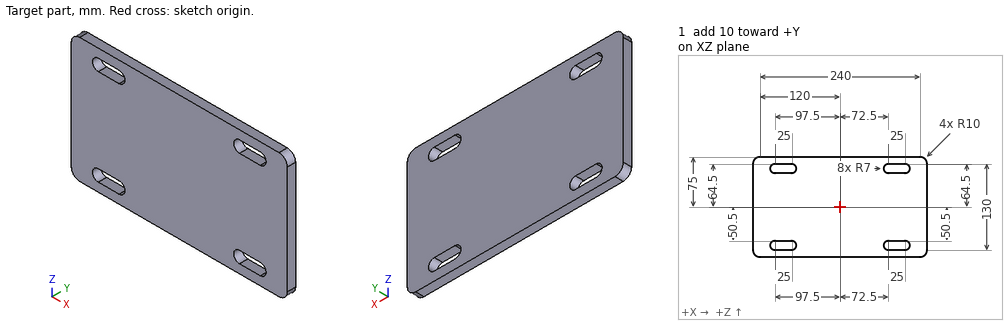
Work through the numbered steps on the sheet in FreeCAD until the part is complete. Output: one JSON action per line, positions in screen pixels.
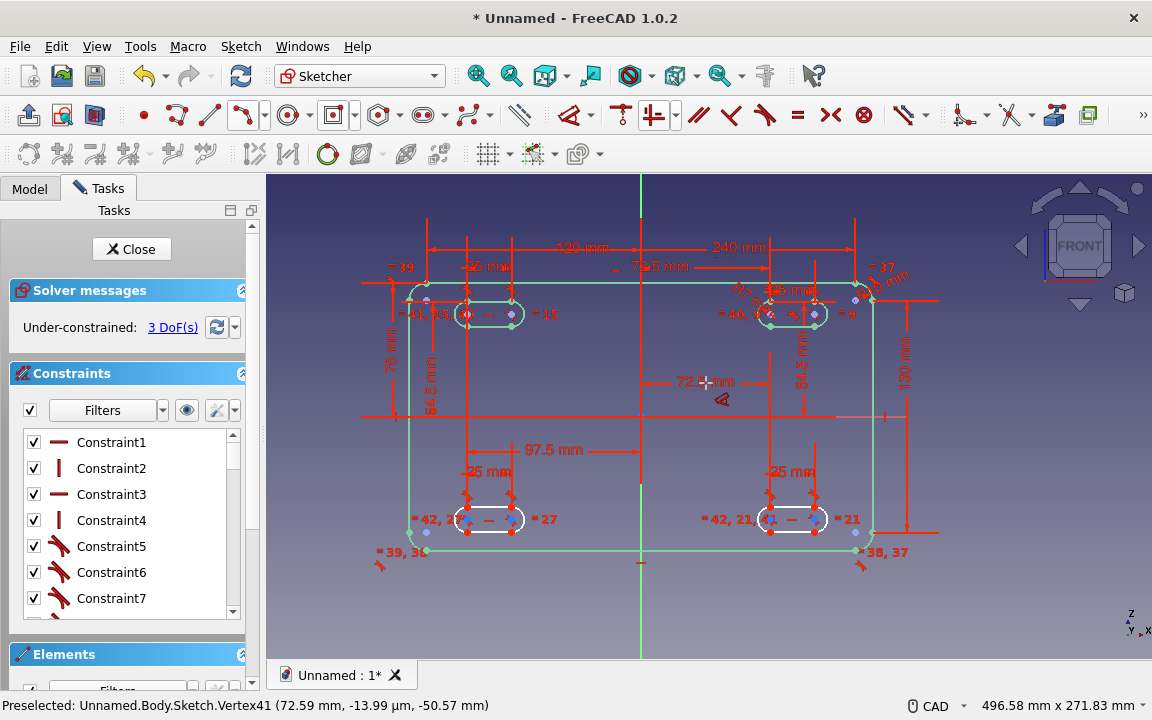
{"action": "left_click", "coordinate": [770, 507]}
{"action": "left_click", "coordinate": [804, 441]}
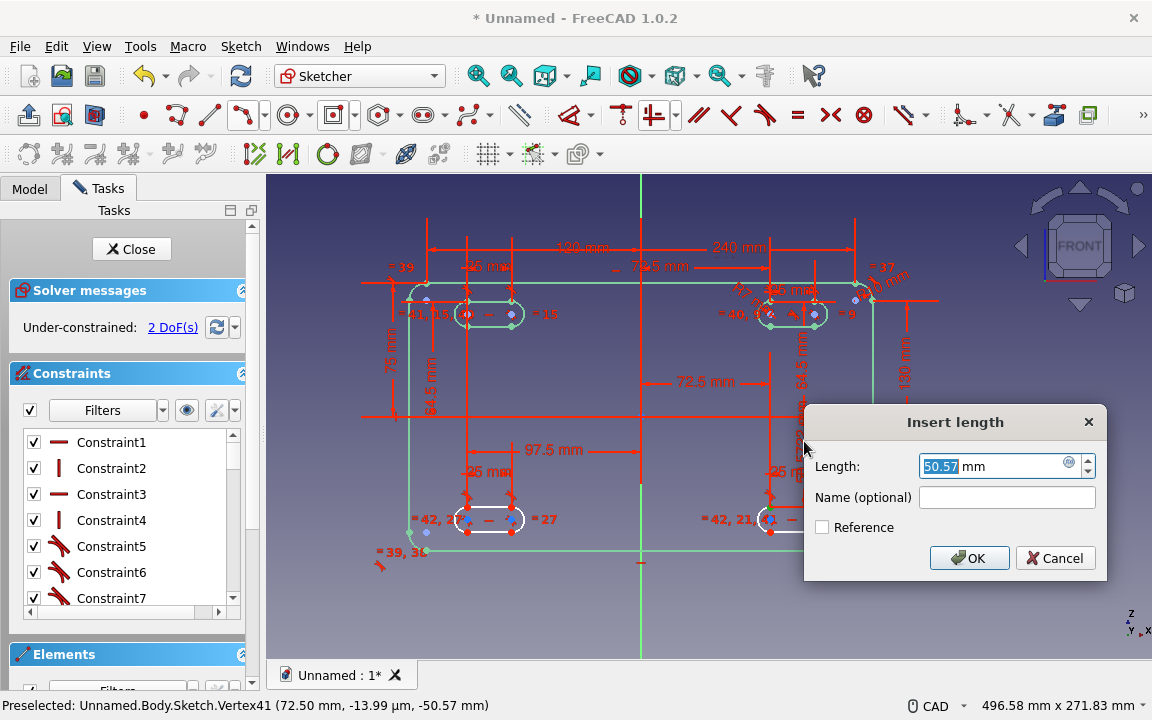
{"action": "type", "text": "50.5"}
{"action": "key", "text": "Return"}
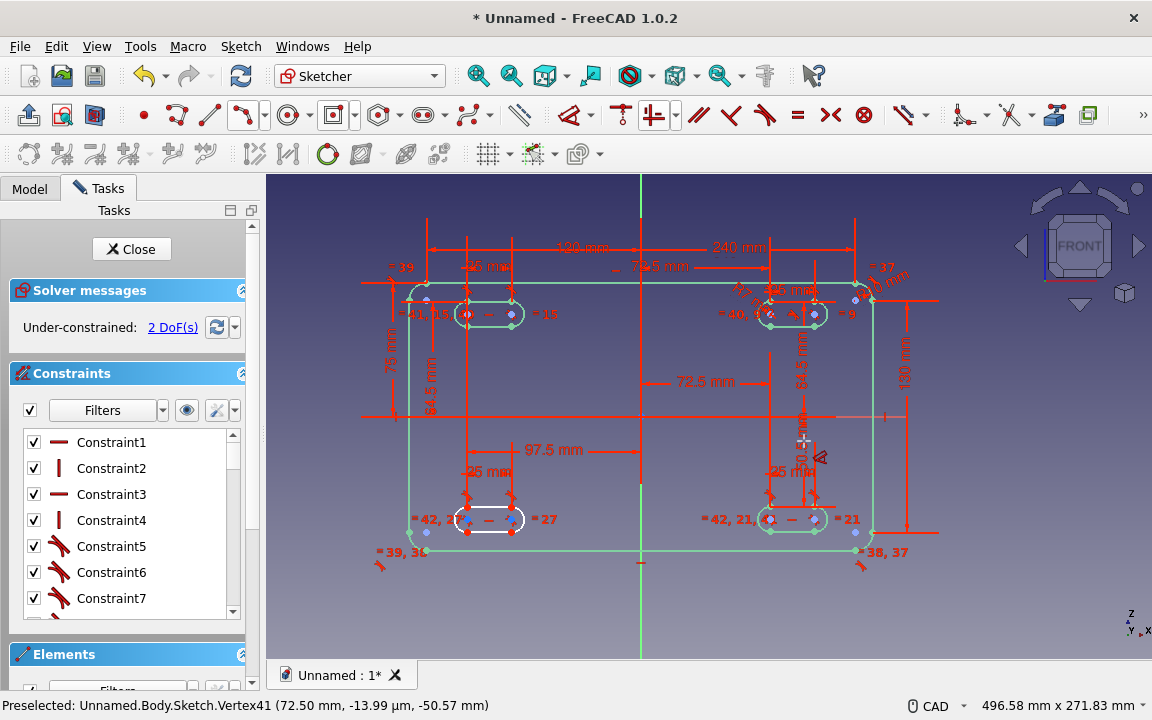
{"action": "left_click", "coordinate": [467, 507]}
{"action": "left_click", "coordinate": [554, 383]}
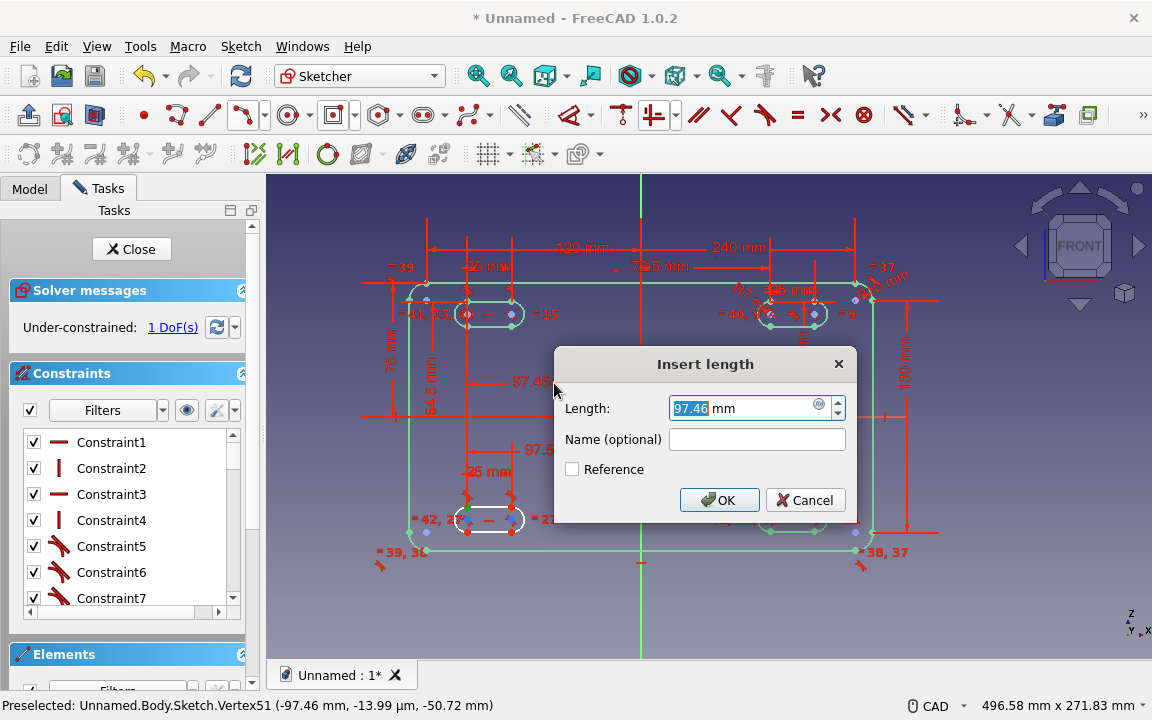
{"action": "type", "text": "97.5"}
{"action": "key", "text": "Return"}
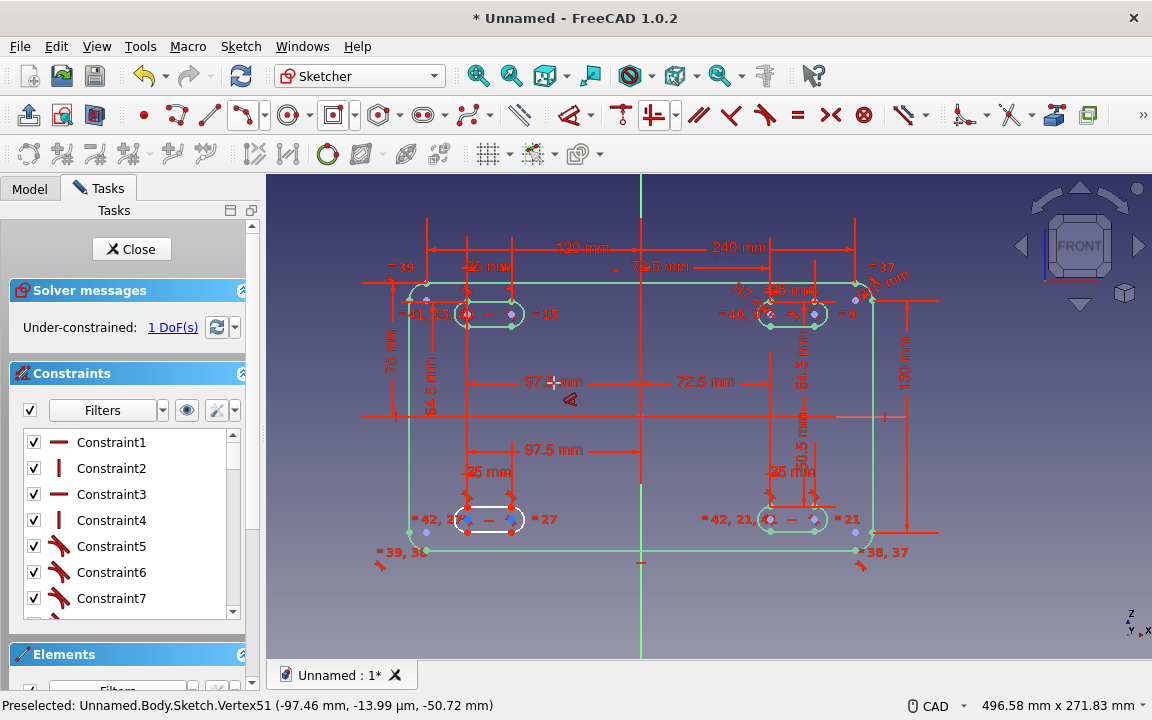
{"action": "left_click", "coordinate": [467, 507]}
{"action": "left_click", "coordinate": [433, 441]}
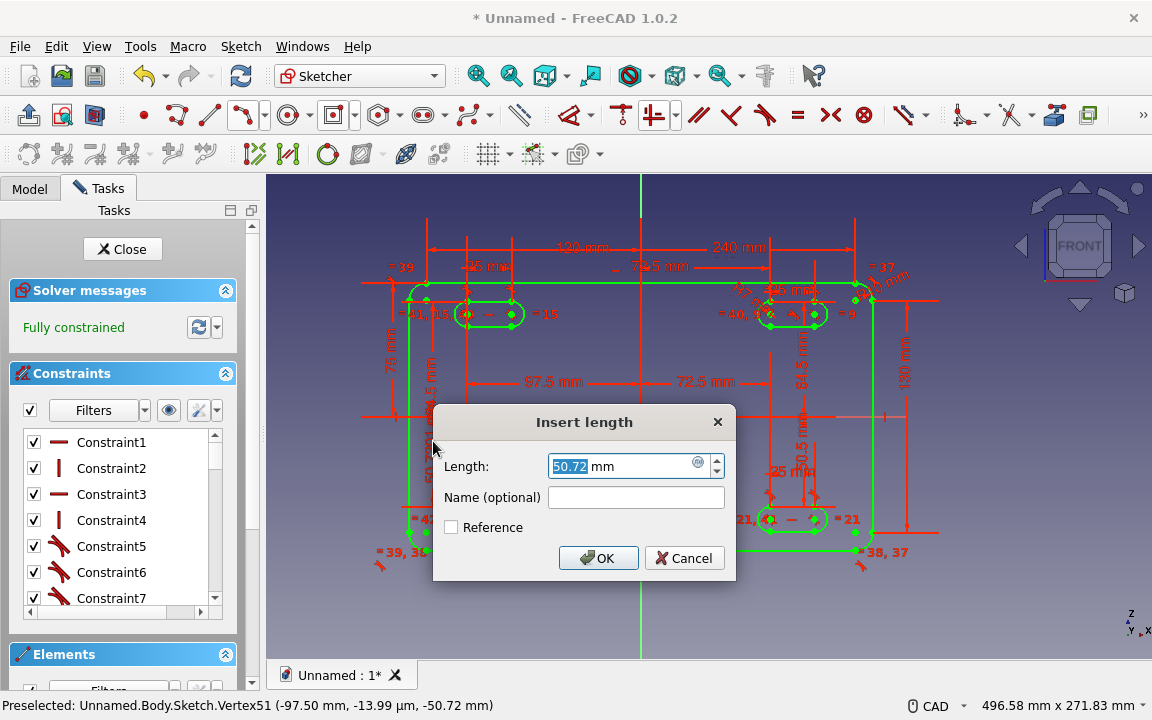
{"action": "type", "text": "50.5"}
{"action": "key", "text": "Return"}
{"action": "key", "text": "Escape"}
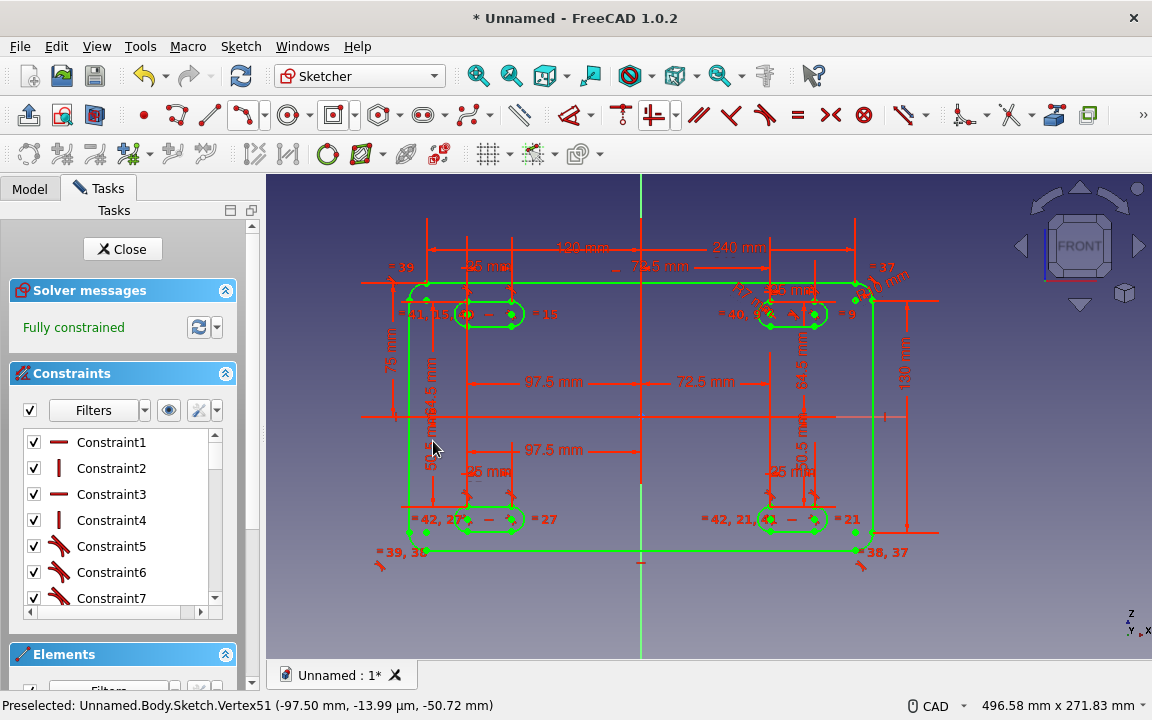
{"action": "left_click", "coordinate": [123, 249]}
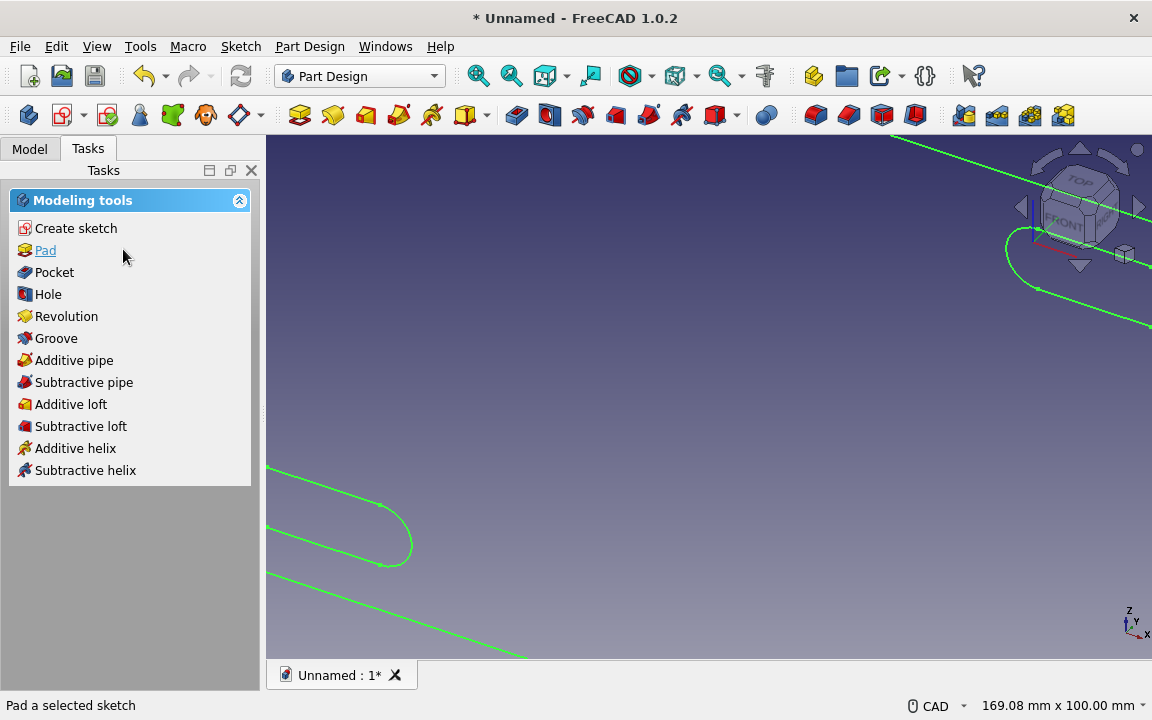
{"action": "left_click", "coordinate": [300, 116]}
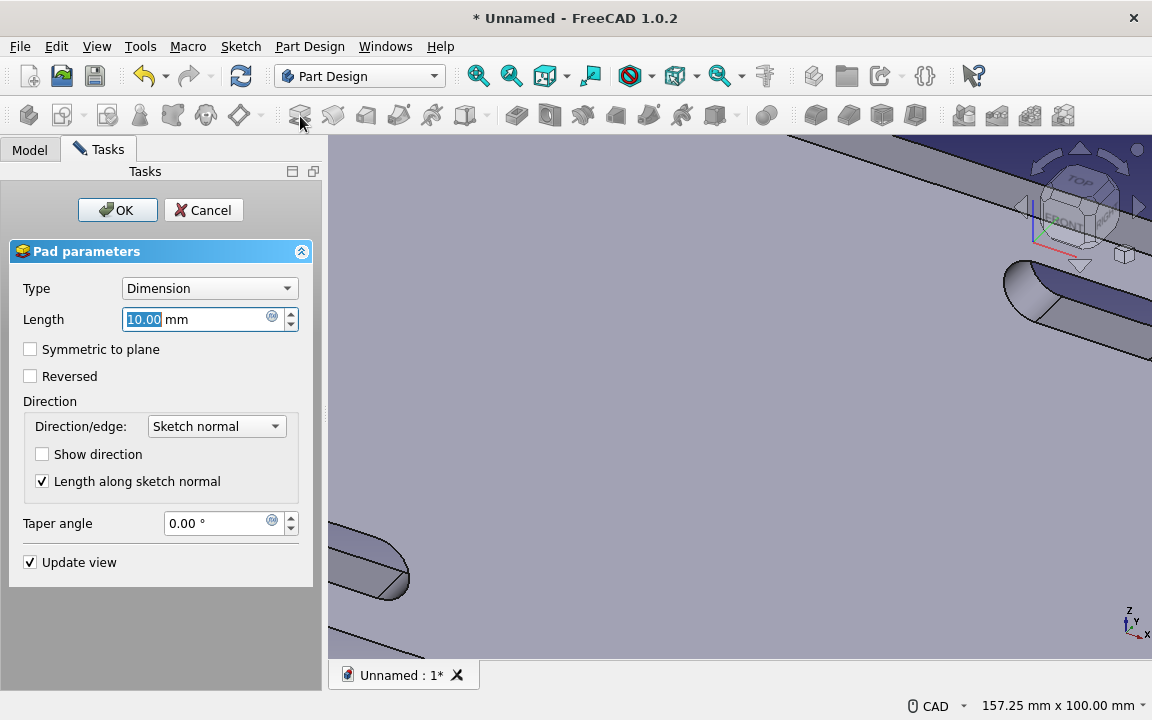
{"action": "type", "text": "10"}
{"action": "key", "text": "Tab"}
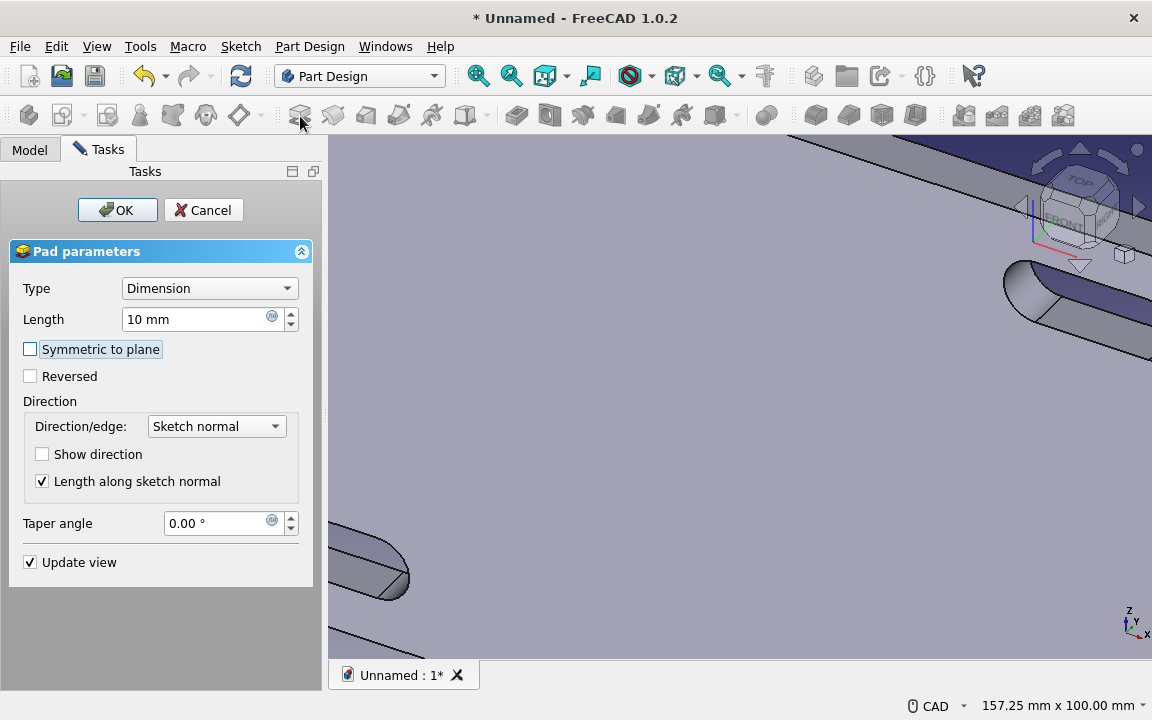
{"action": "left_click", "coordinate": [31, 376]}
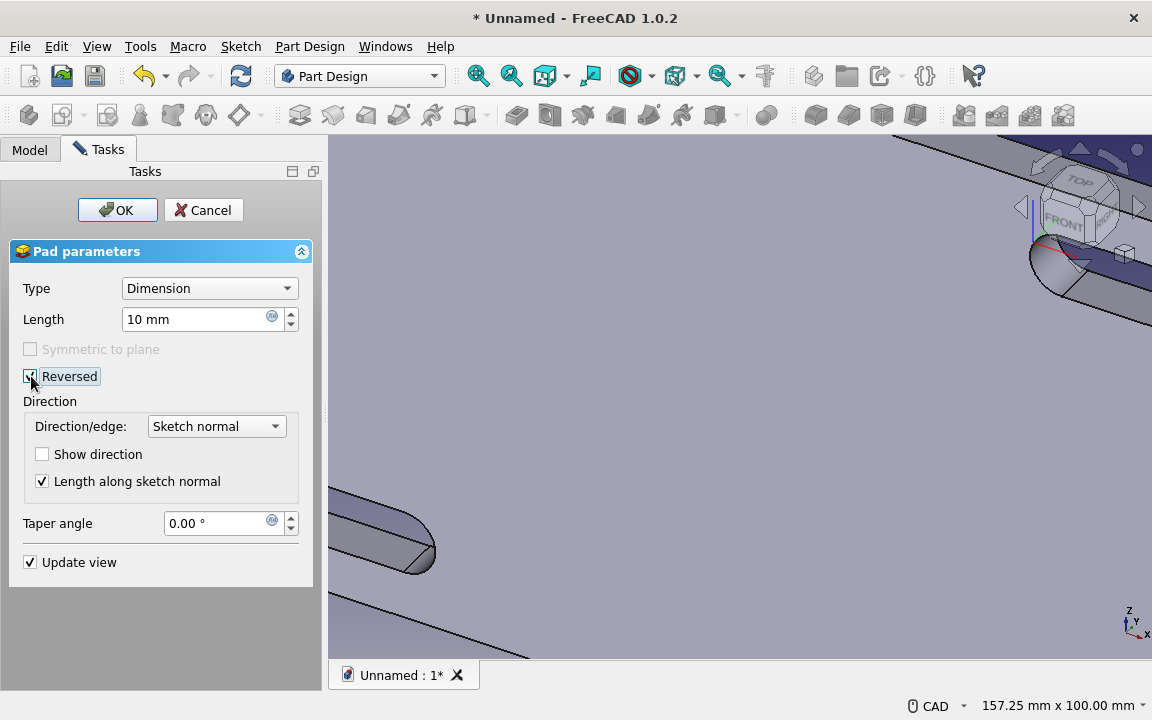
{"action": "left_click", "coordinate": [118, 210]}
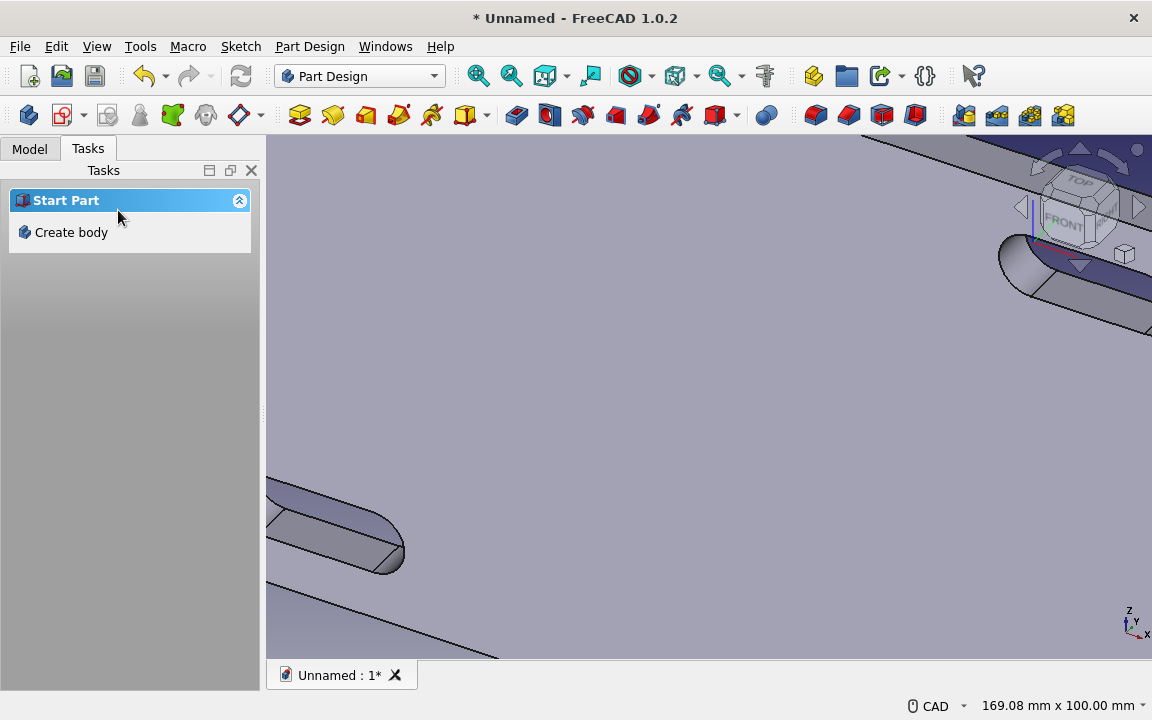
{"action": "key", "text": "0"}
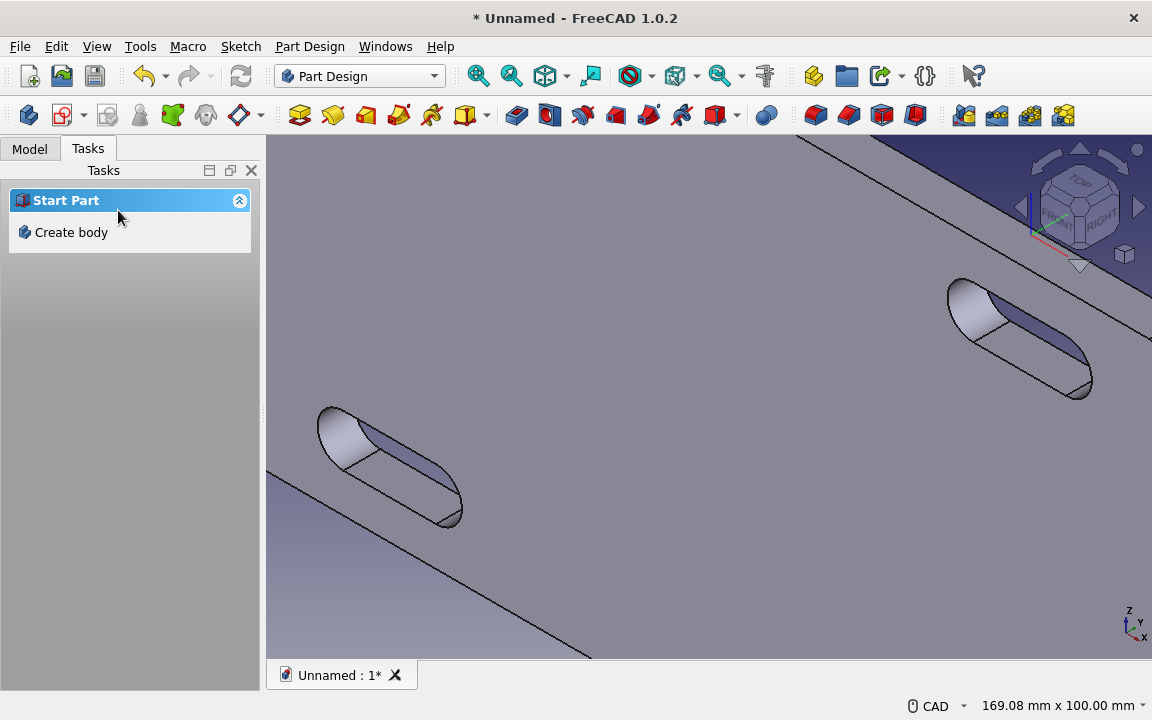
{"action": "left_click", "coordinate": [479, 76]}